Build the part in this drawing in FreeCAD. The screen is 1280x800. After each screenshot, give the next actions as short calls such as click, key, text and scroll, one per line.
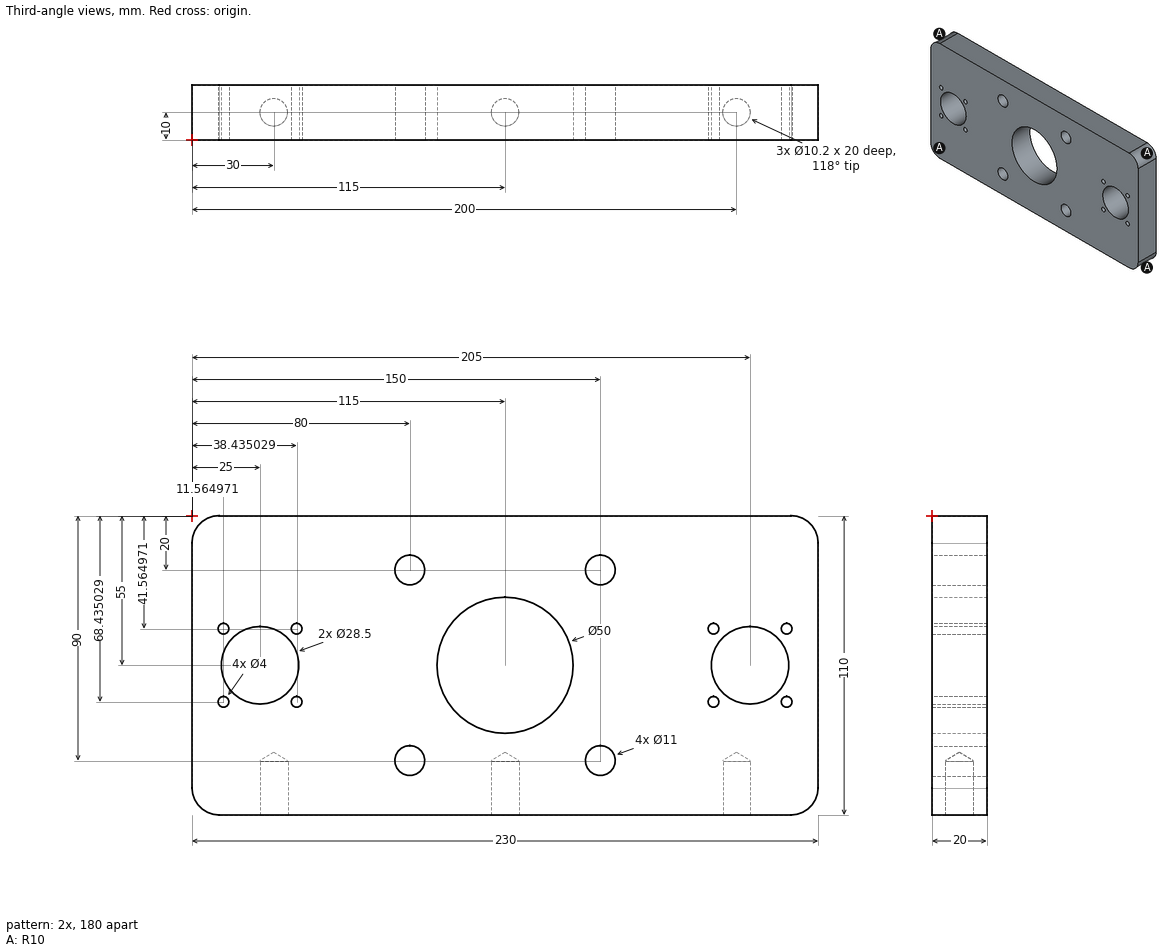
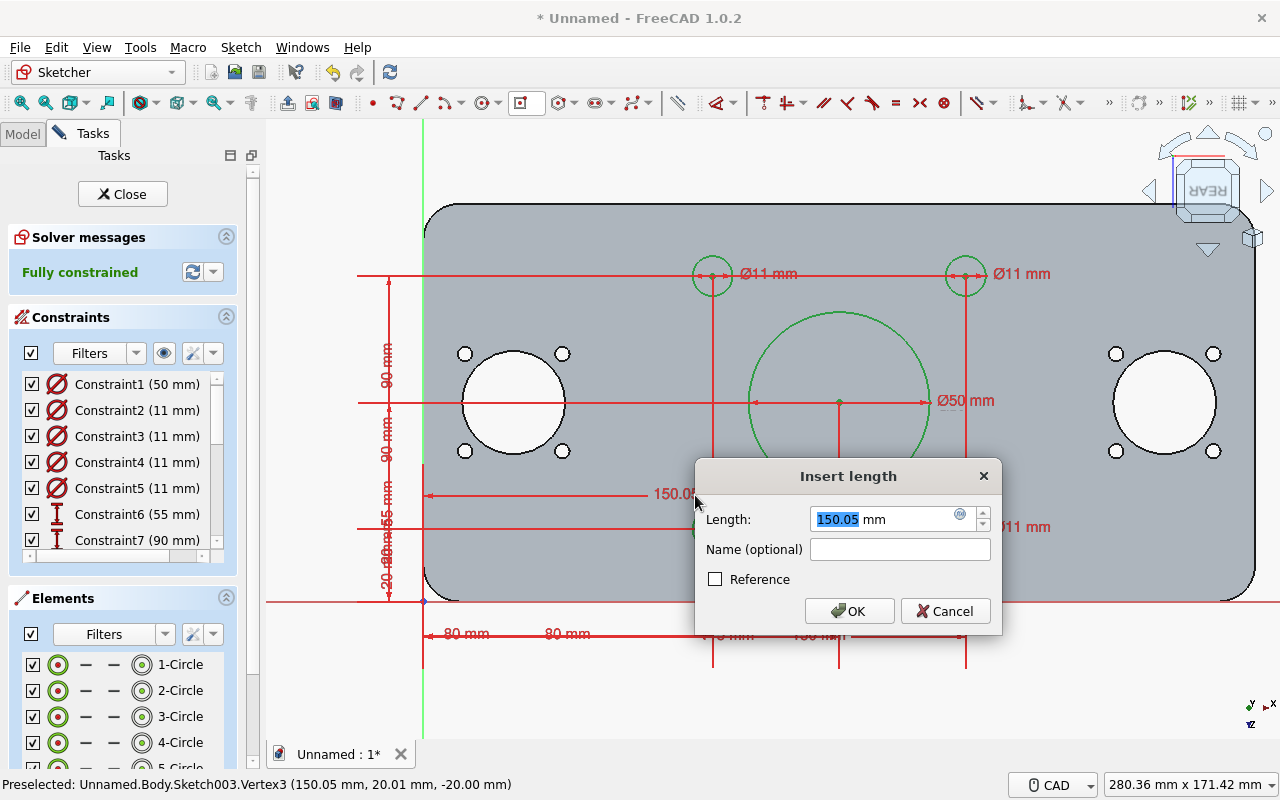
text(150)
key(Return)
key(Escape)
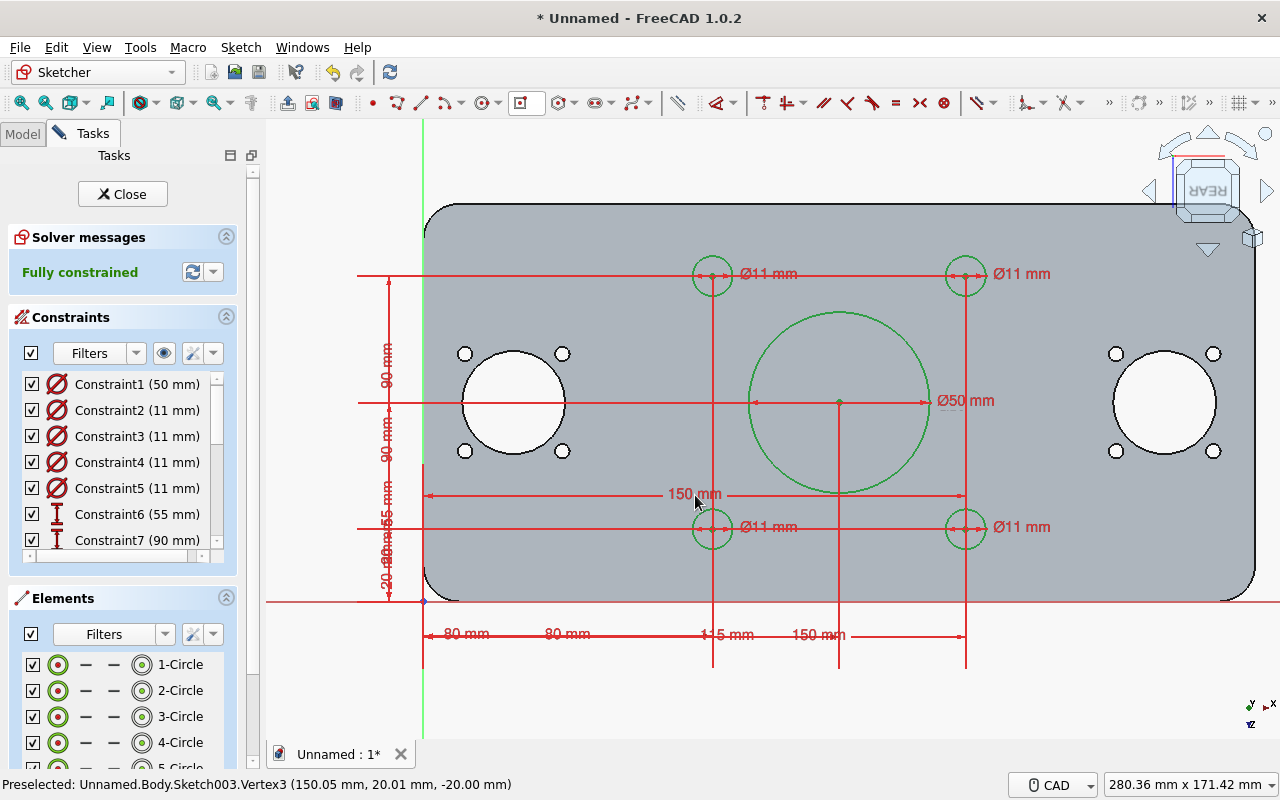
click(123, 194)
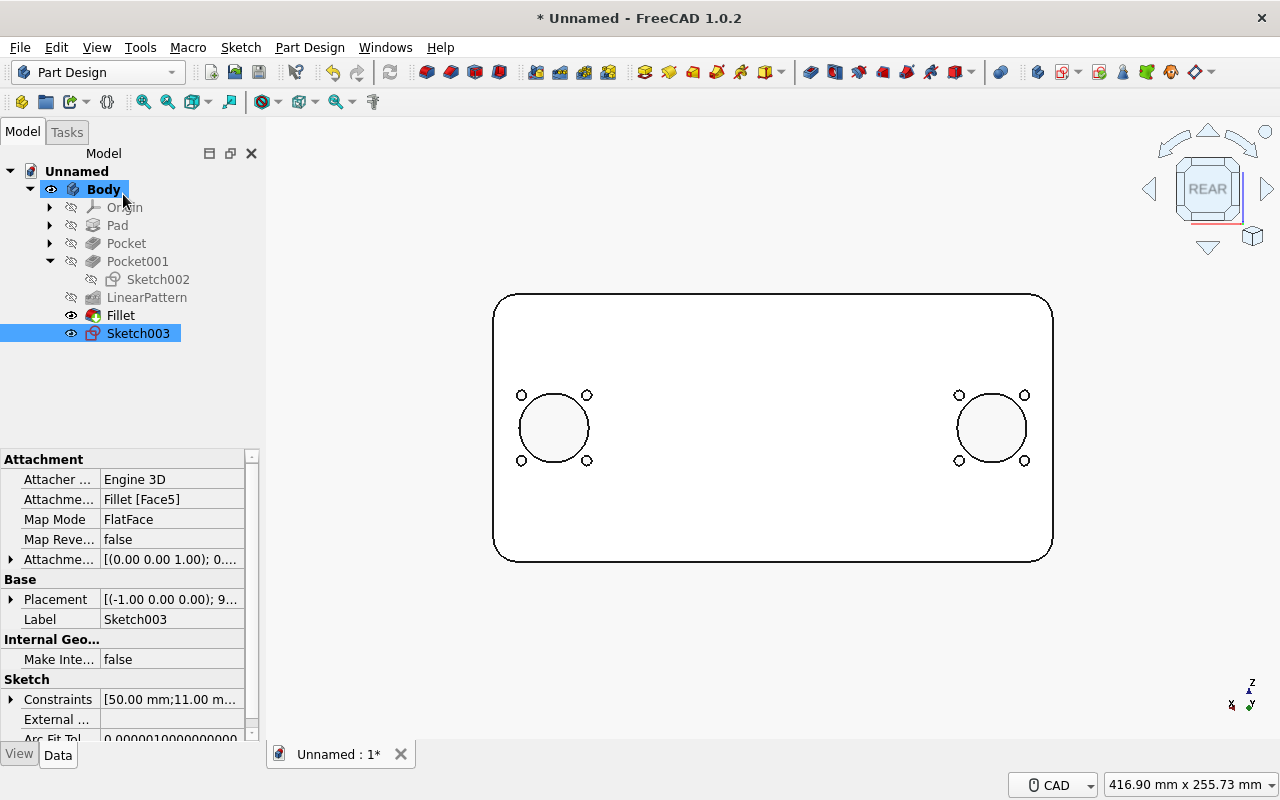
click(812, 72)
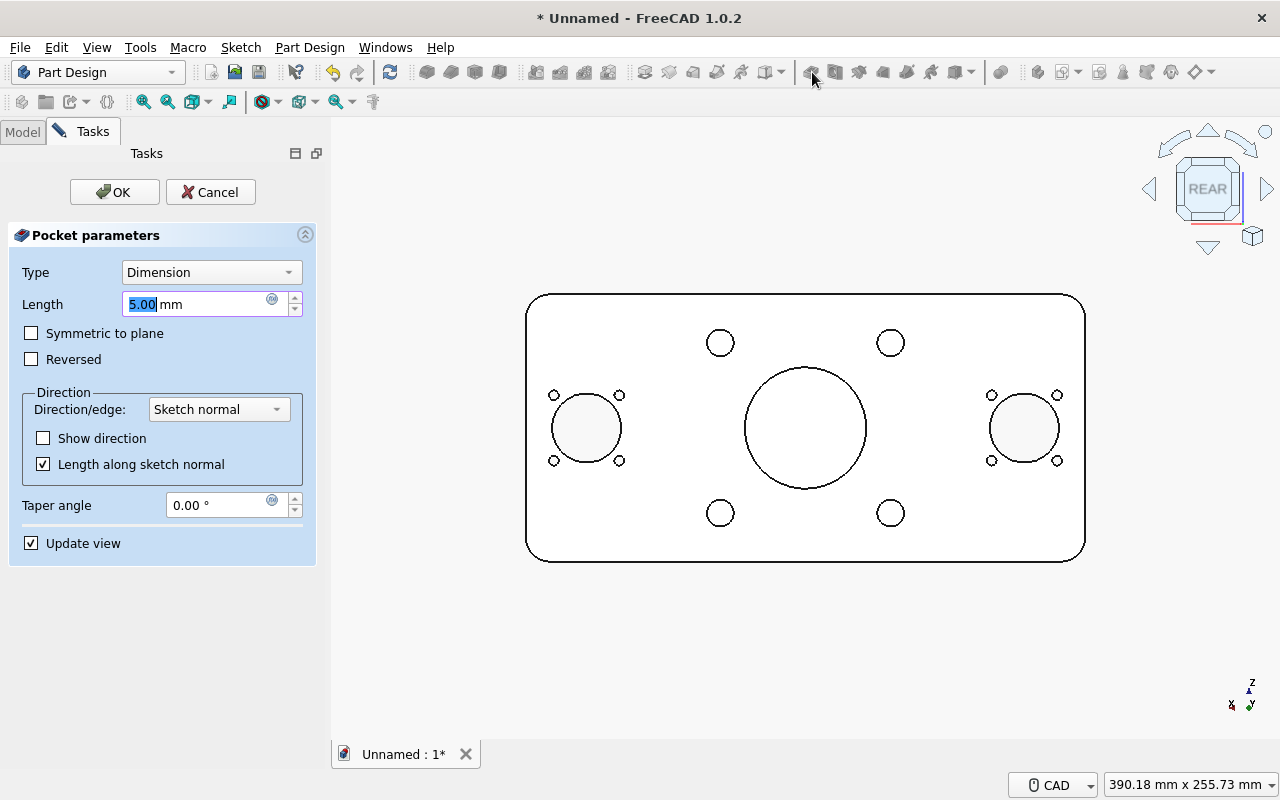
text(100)
key(Tab)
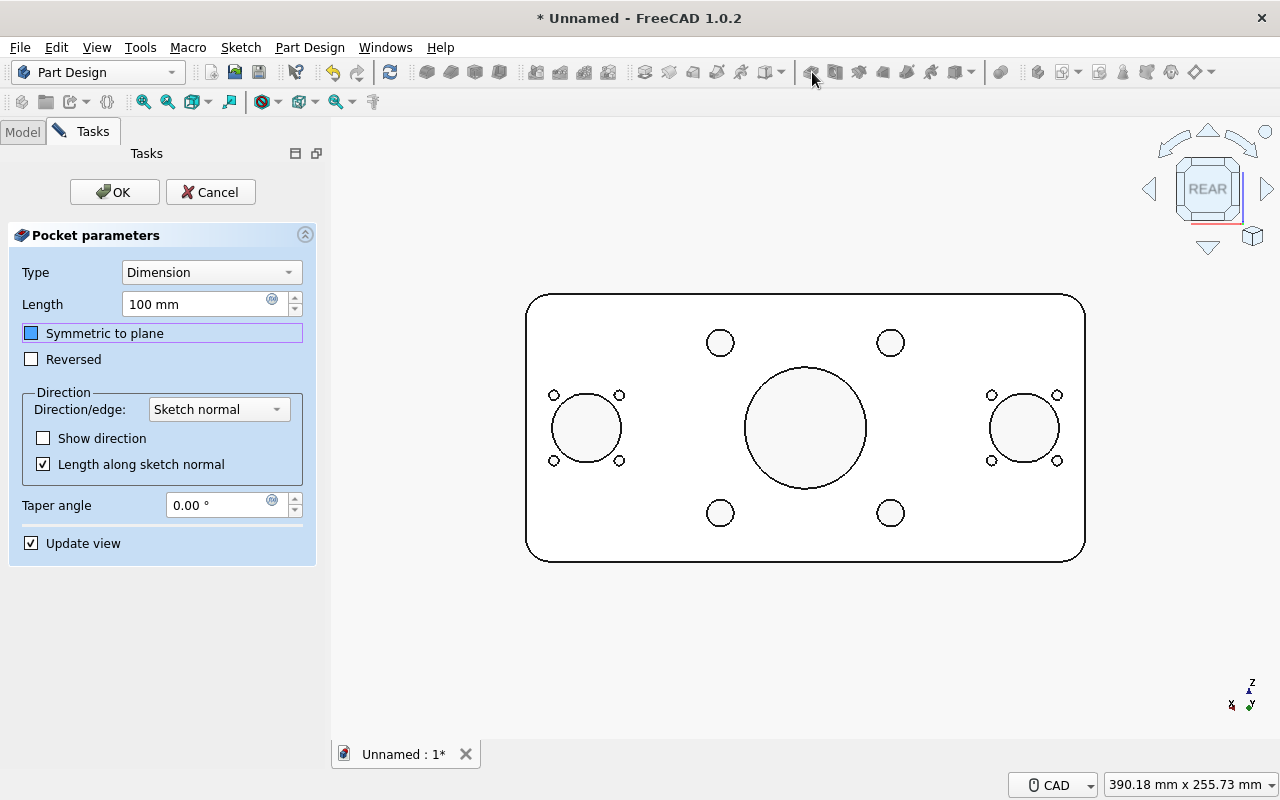
click(115, 192)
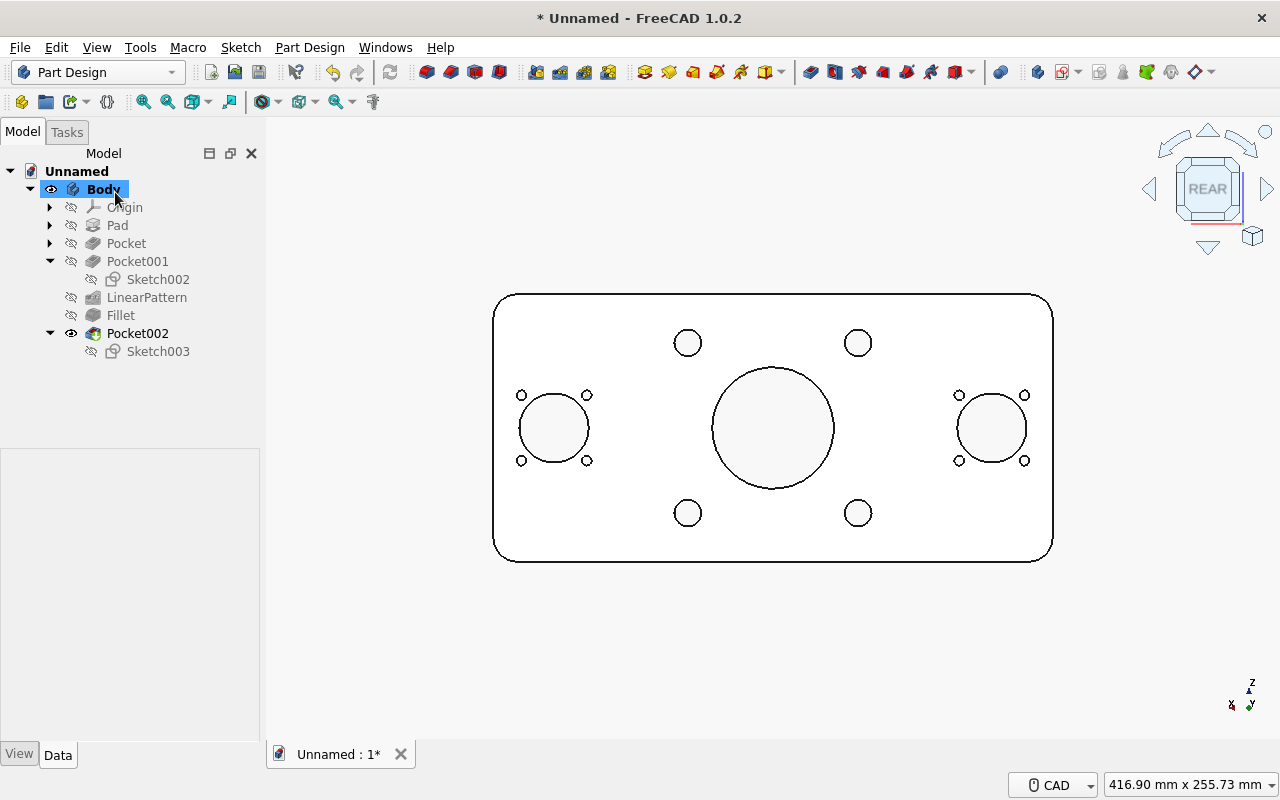
key(5)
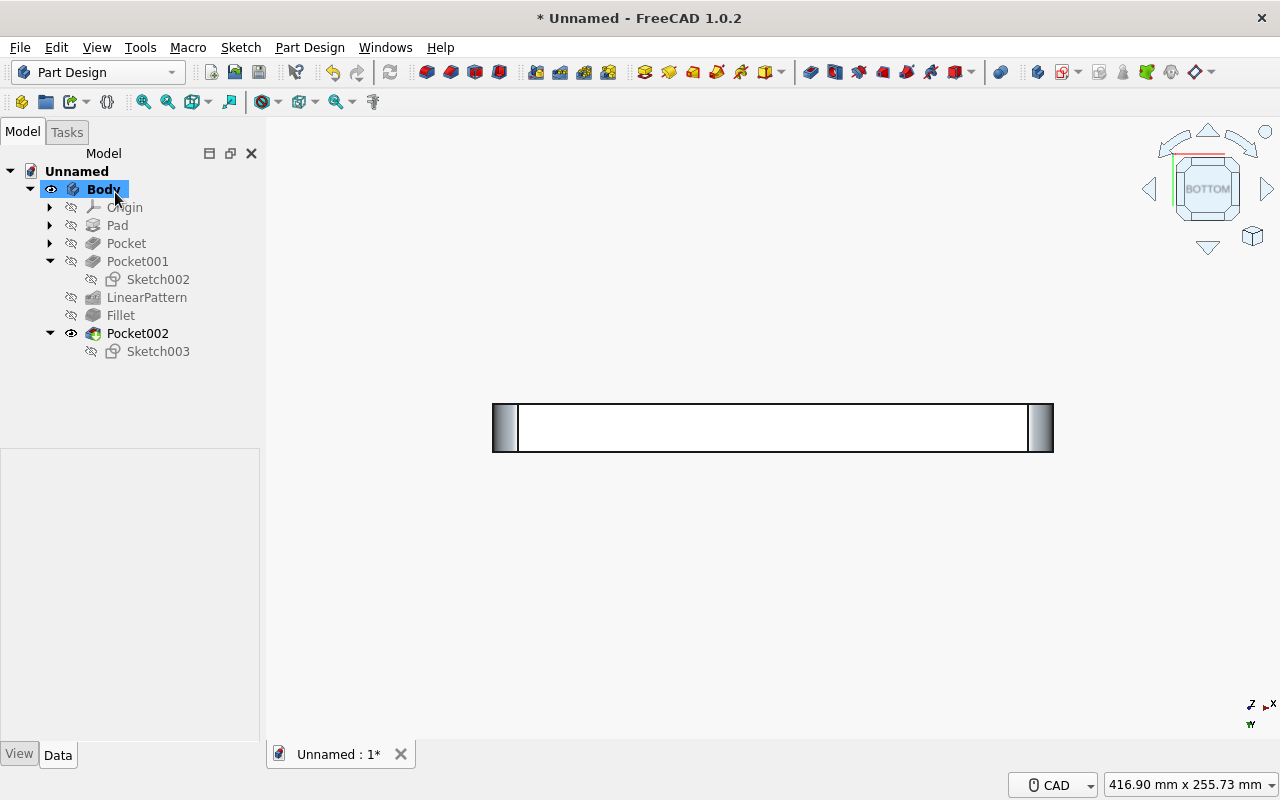
click(992, 427)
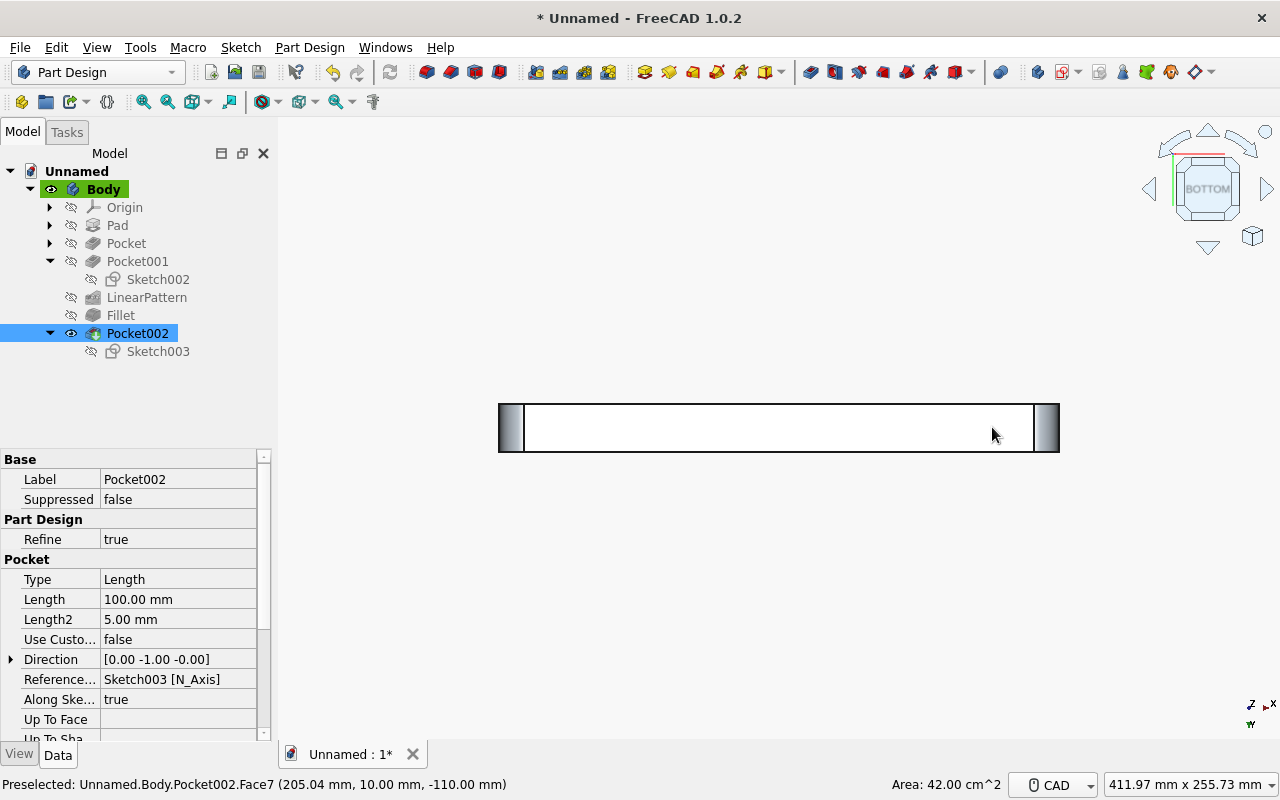
click(1062, 72)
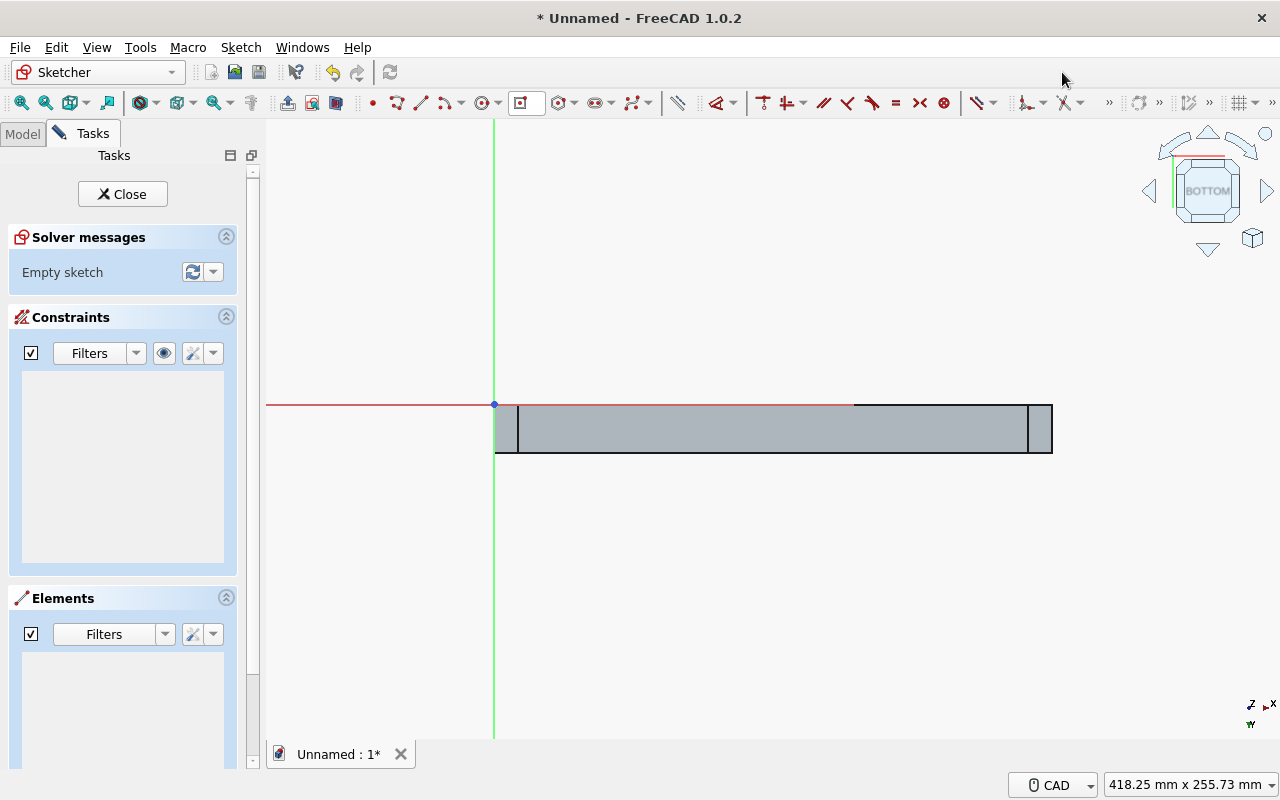
click(482, 104)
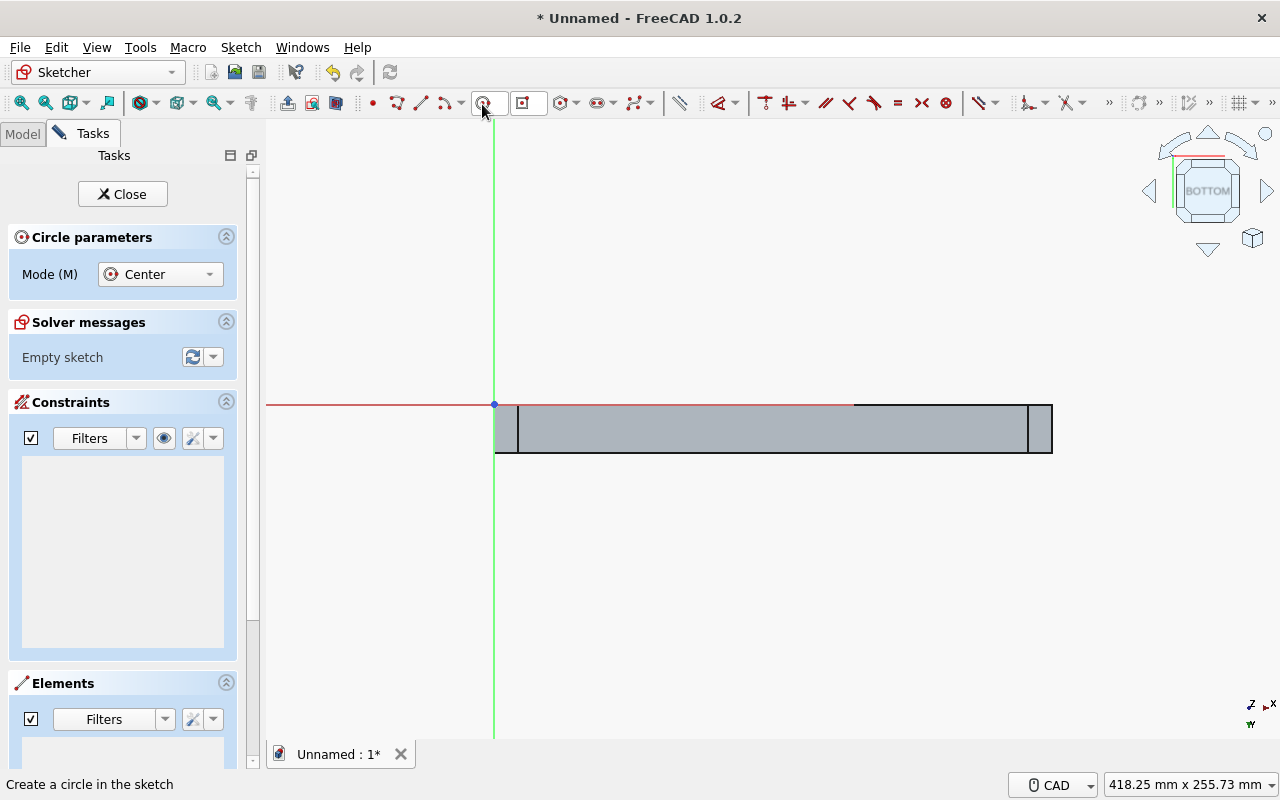
scroll(979, 429, up, 4)